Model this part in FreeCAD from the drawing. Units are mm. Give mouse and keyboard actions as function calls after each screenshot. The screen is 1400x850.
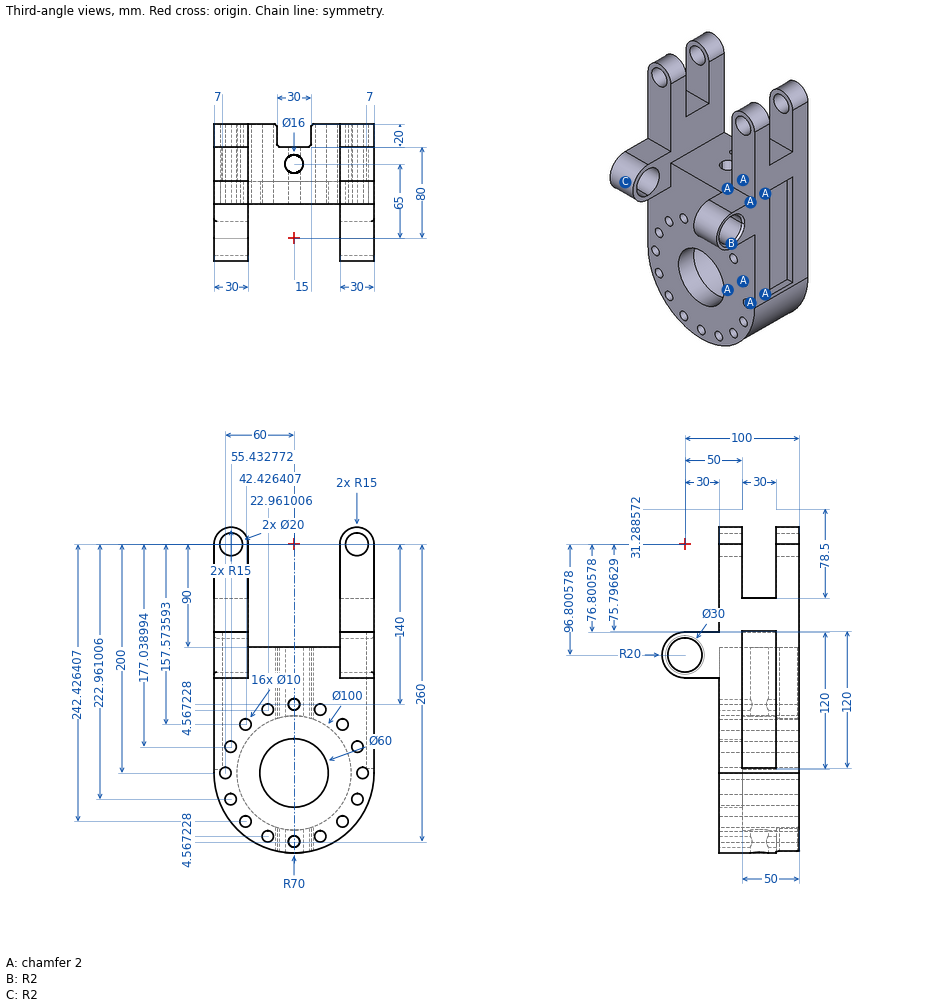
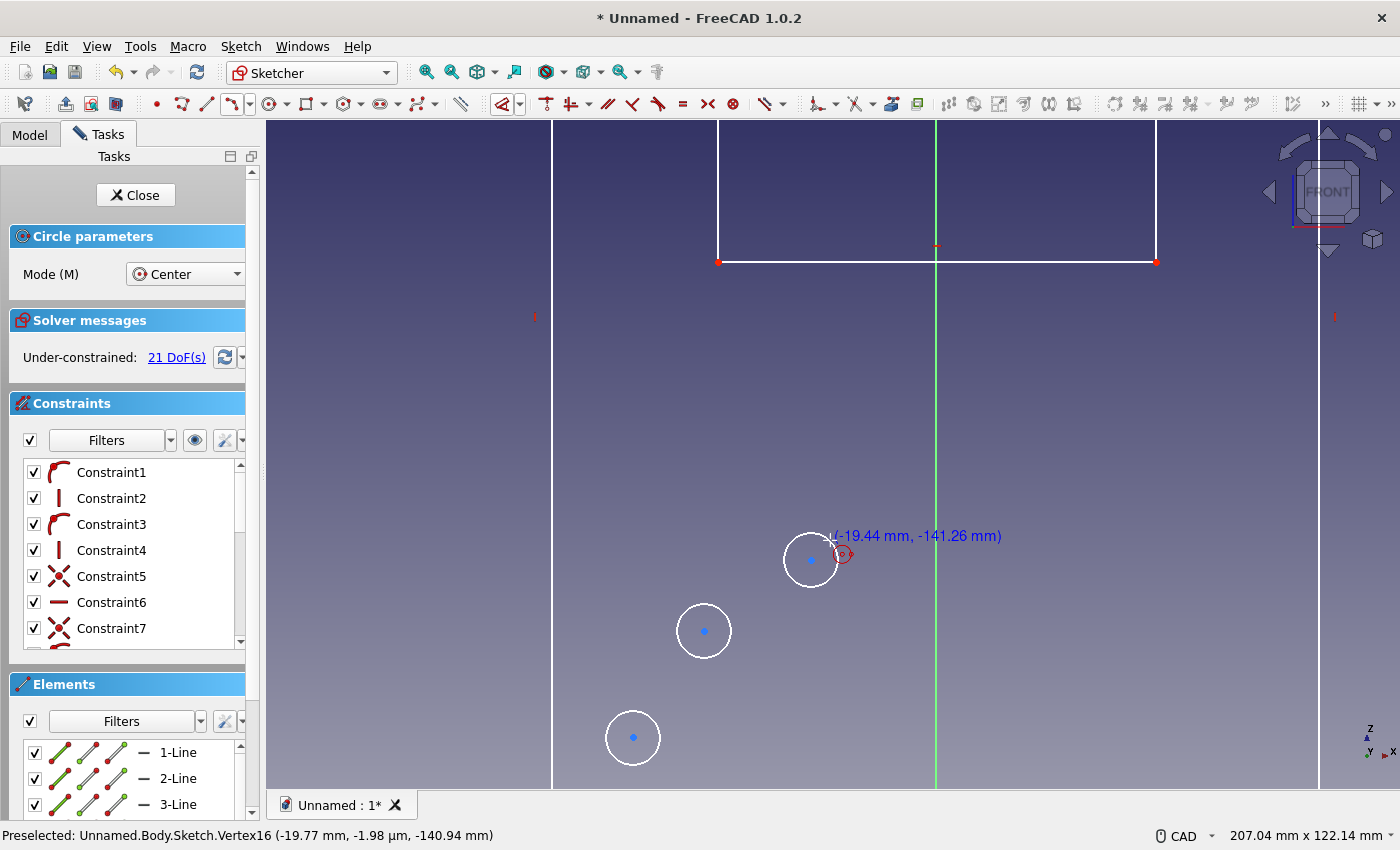
scroll(690, 450, down, 6)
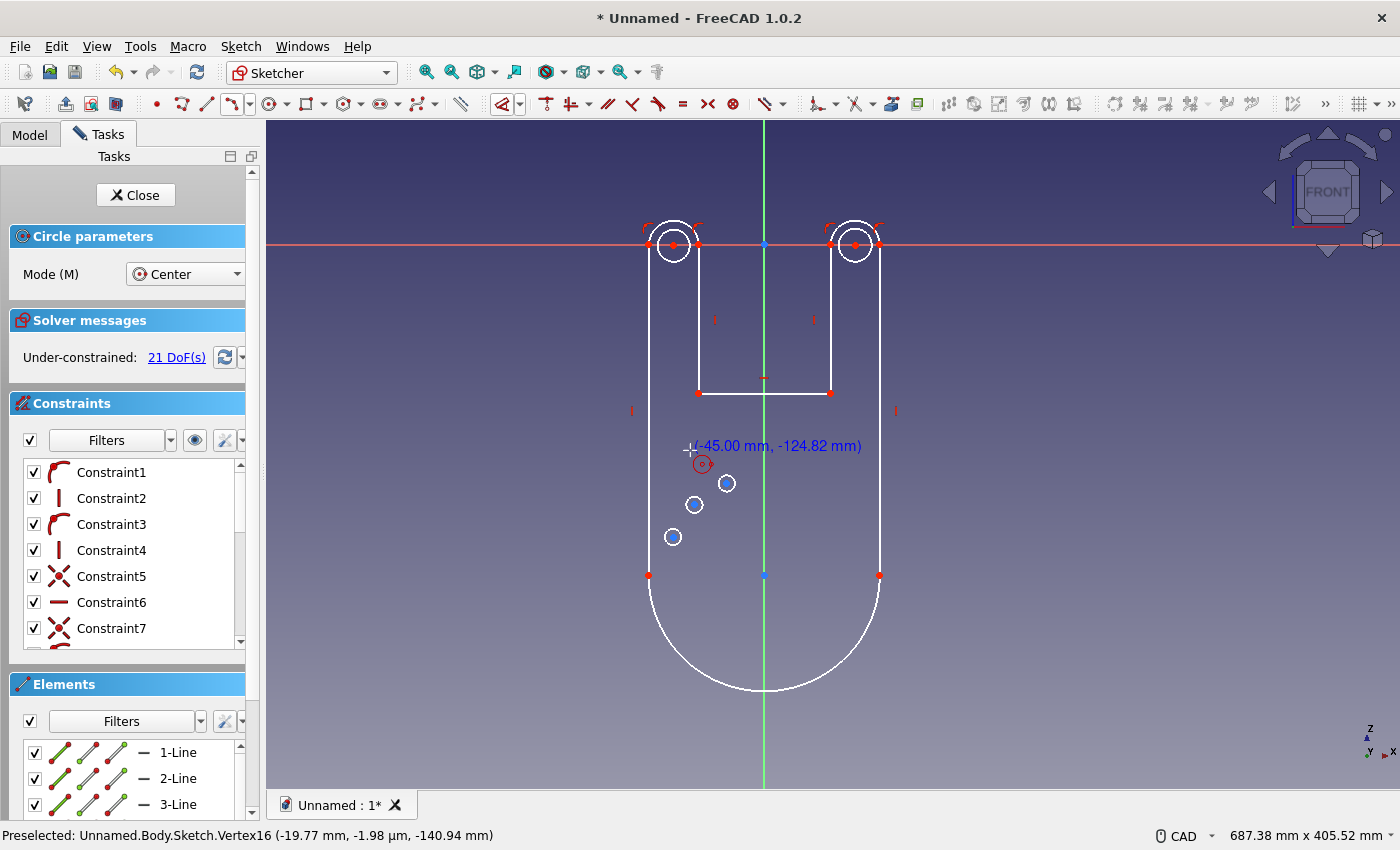
scroll(666, 575, up, 6)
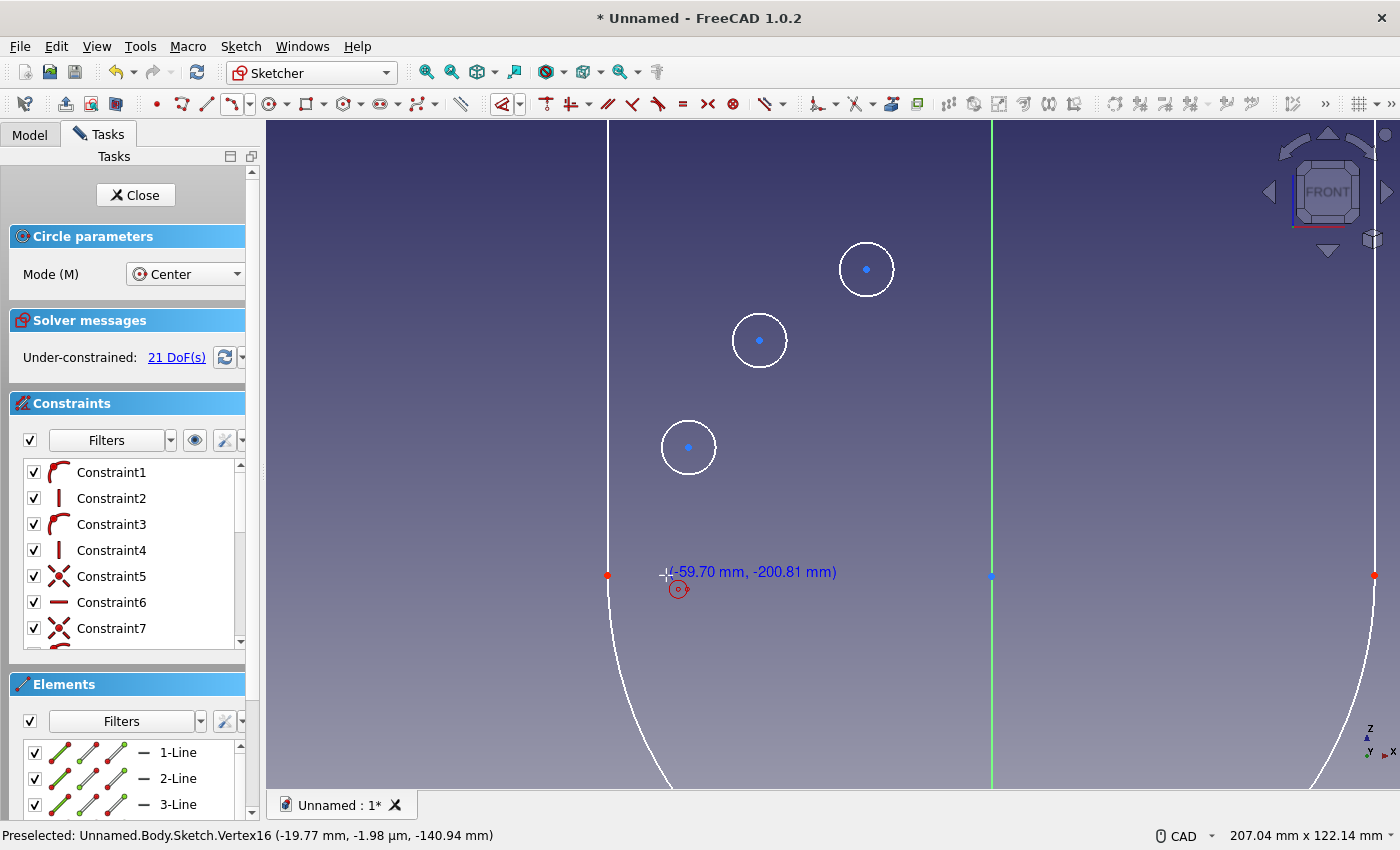
click(664, 572)
click(683, 553)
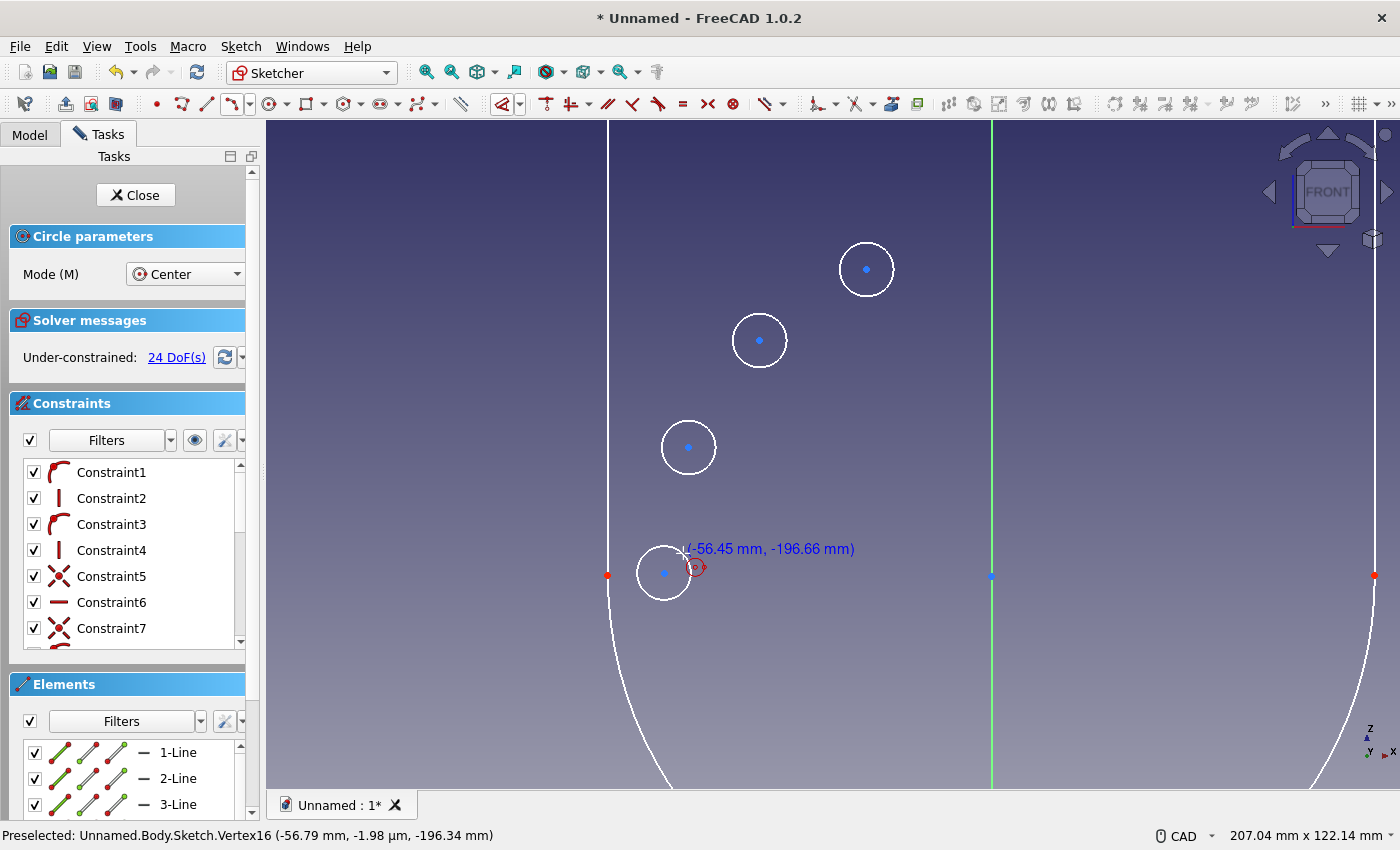
click(689, 698)
click(708, 679)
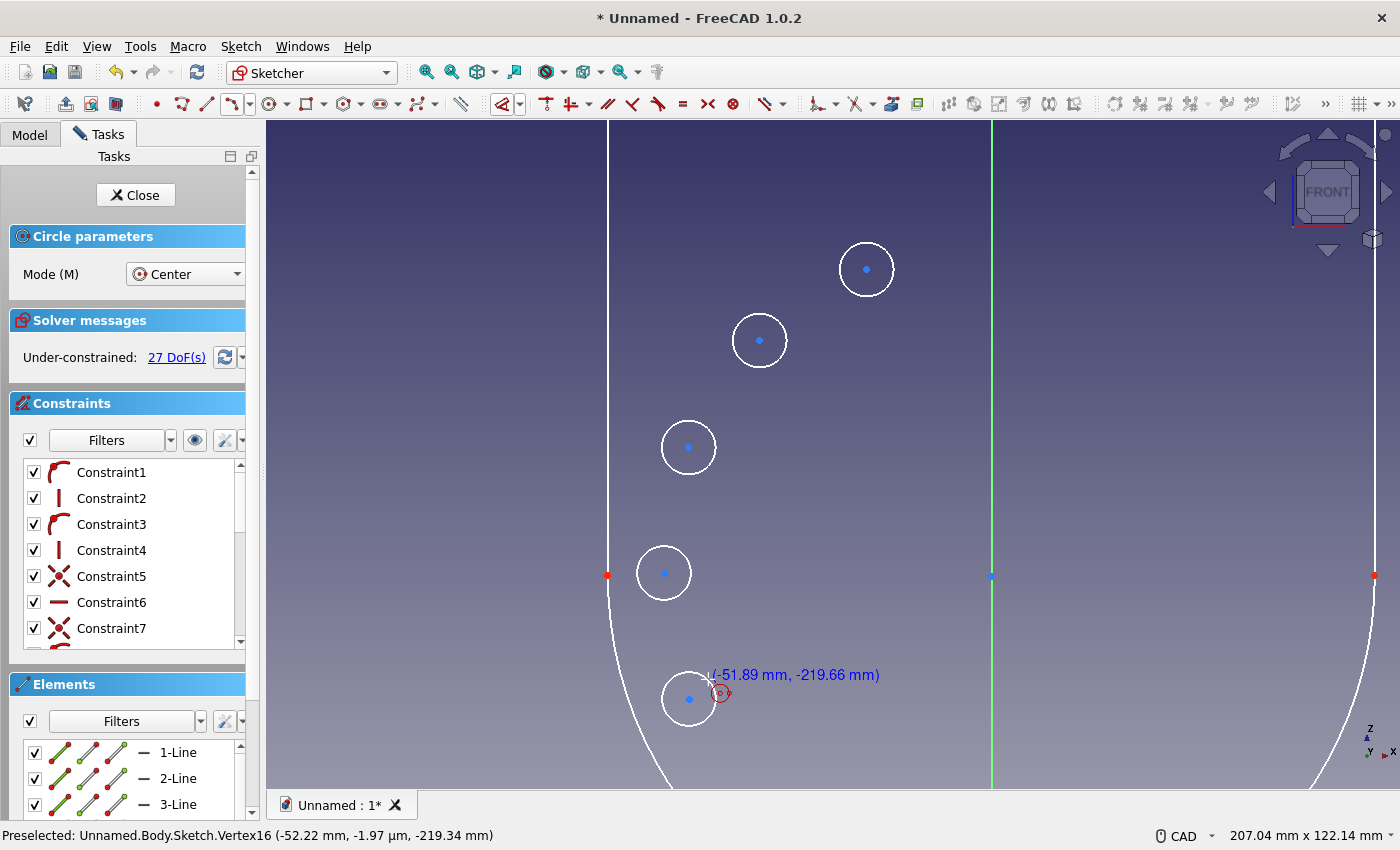
scroll(666, 575, down, 6)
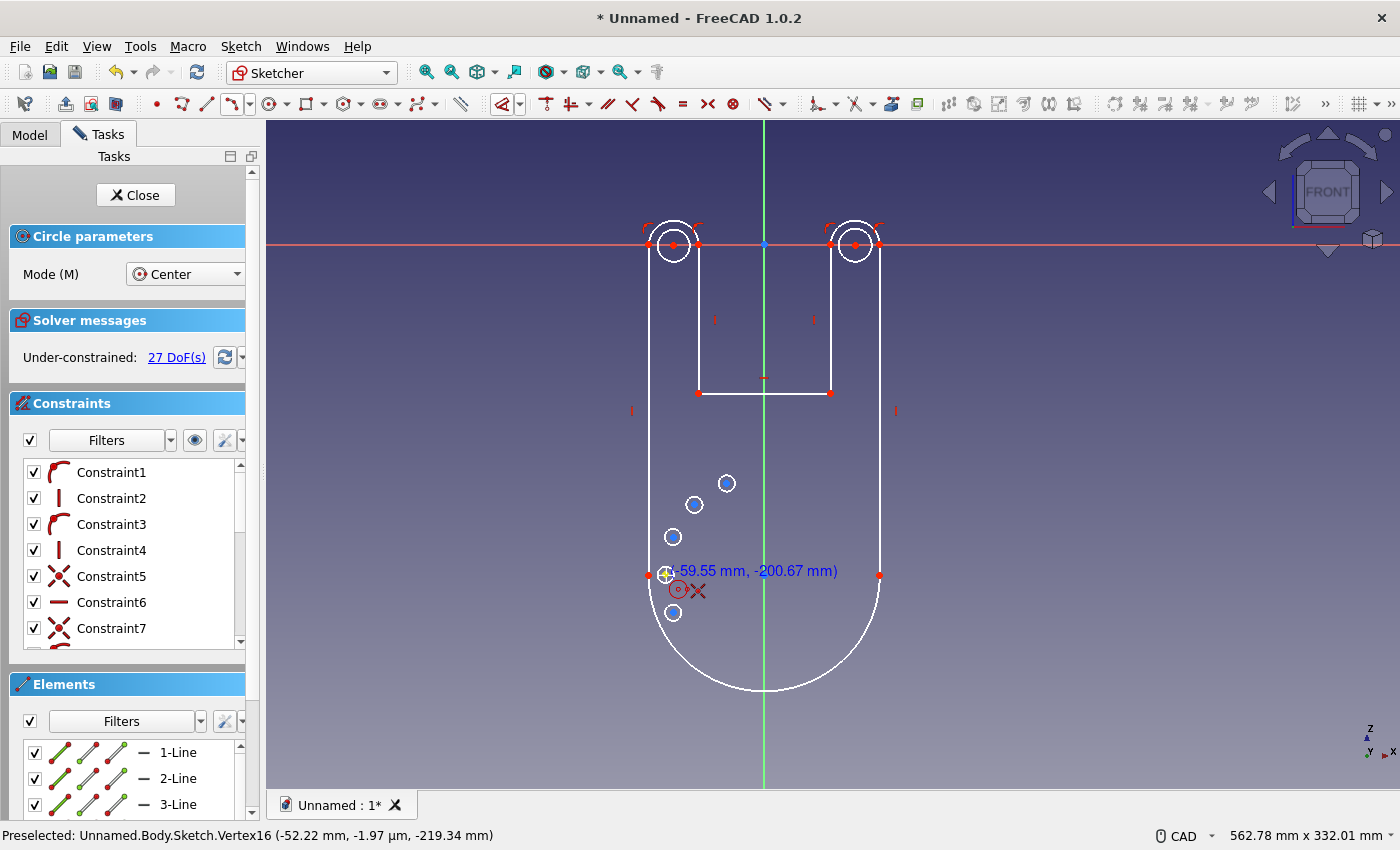
scroll(695, 645, up, 6)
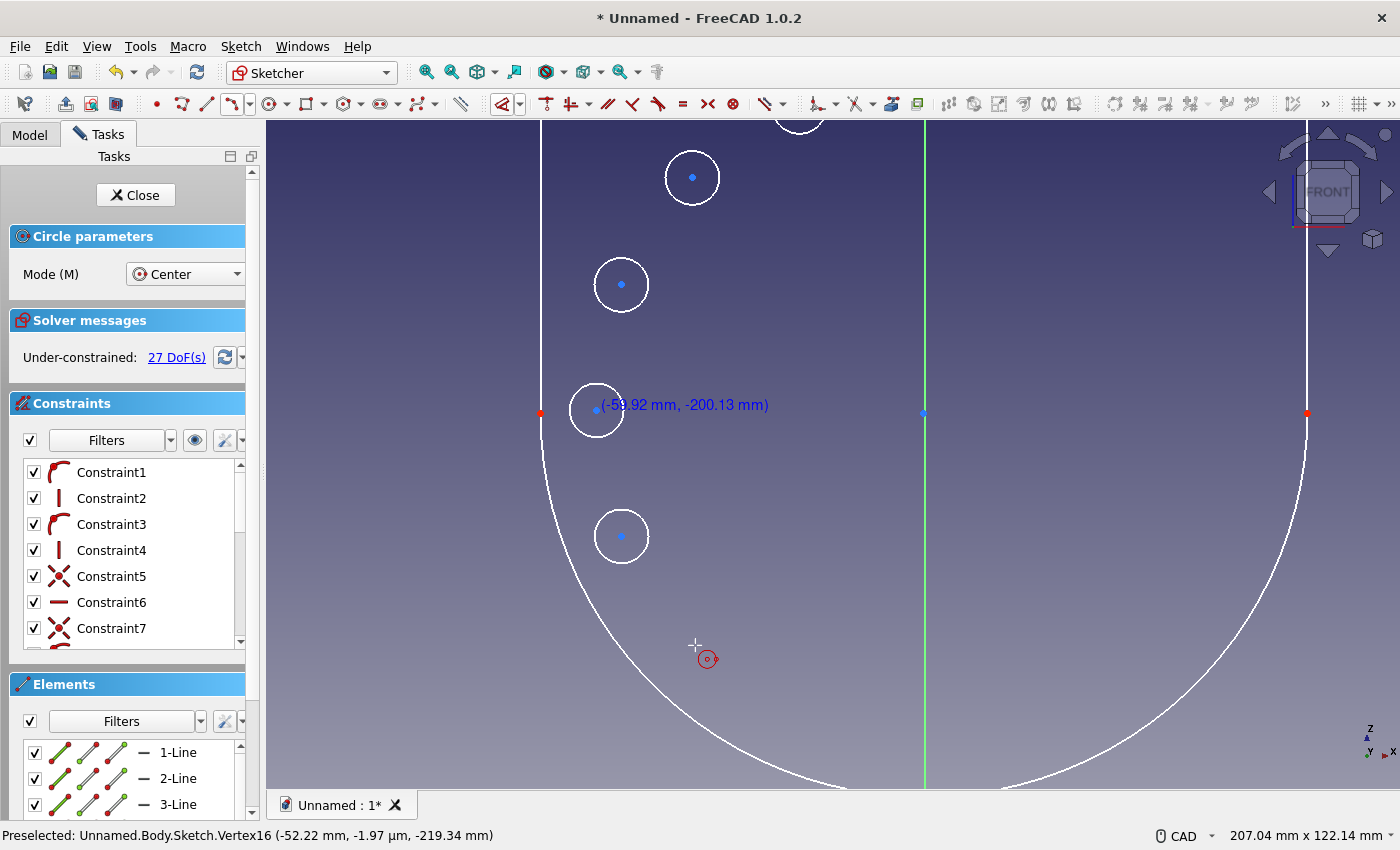
click(692, 642)
click(712, 623)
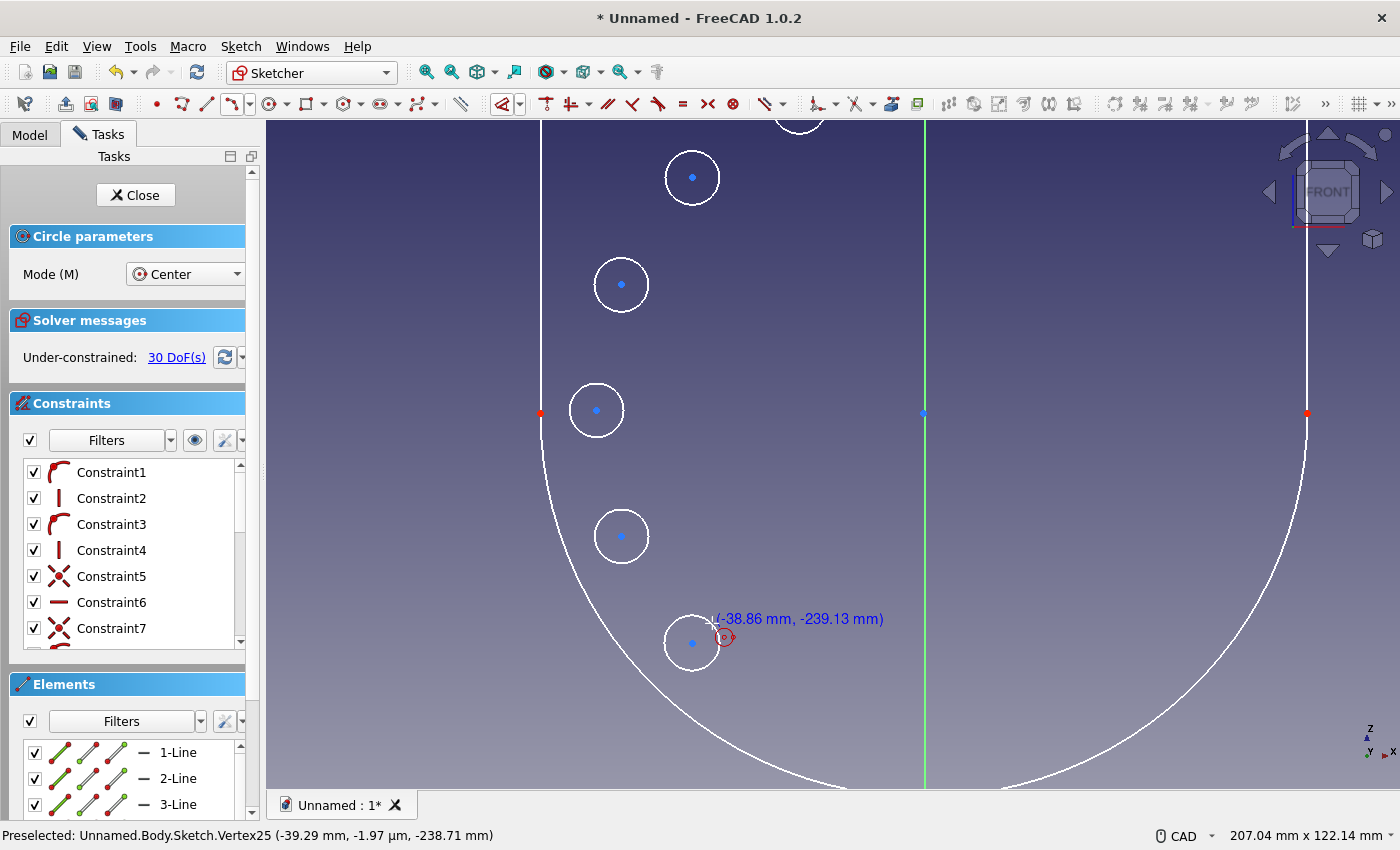
click(799, 713)
click(818, 694)